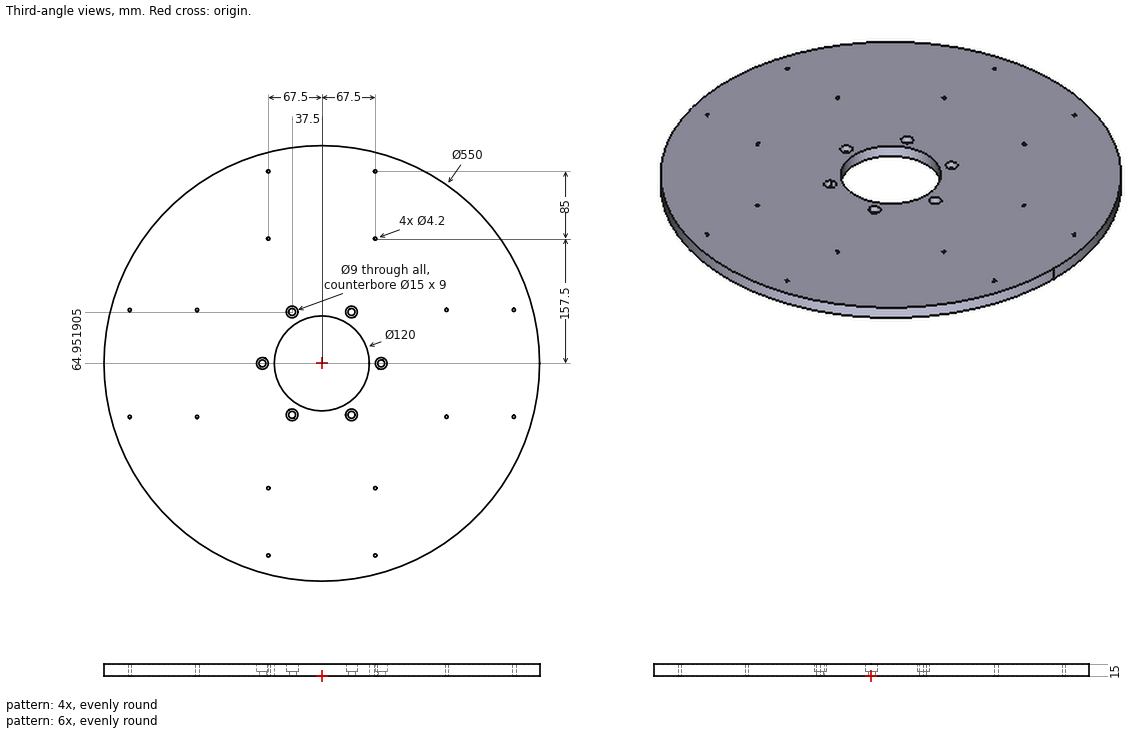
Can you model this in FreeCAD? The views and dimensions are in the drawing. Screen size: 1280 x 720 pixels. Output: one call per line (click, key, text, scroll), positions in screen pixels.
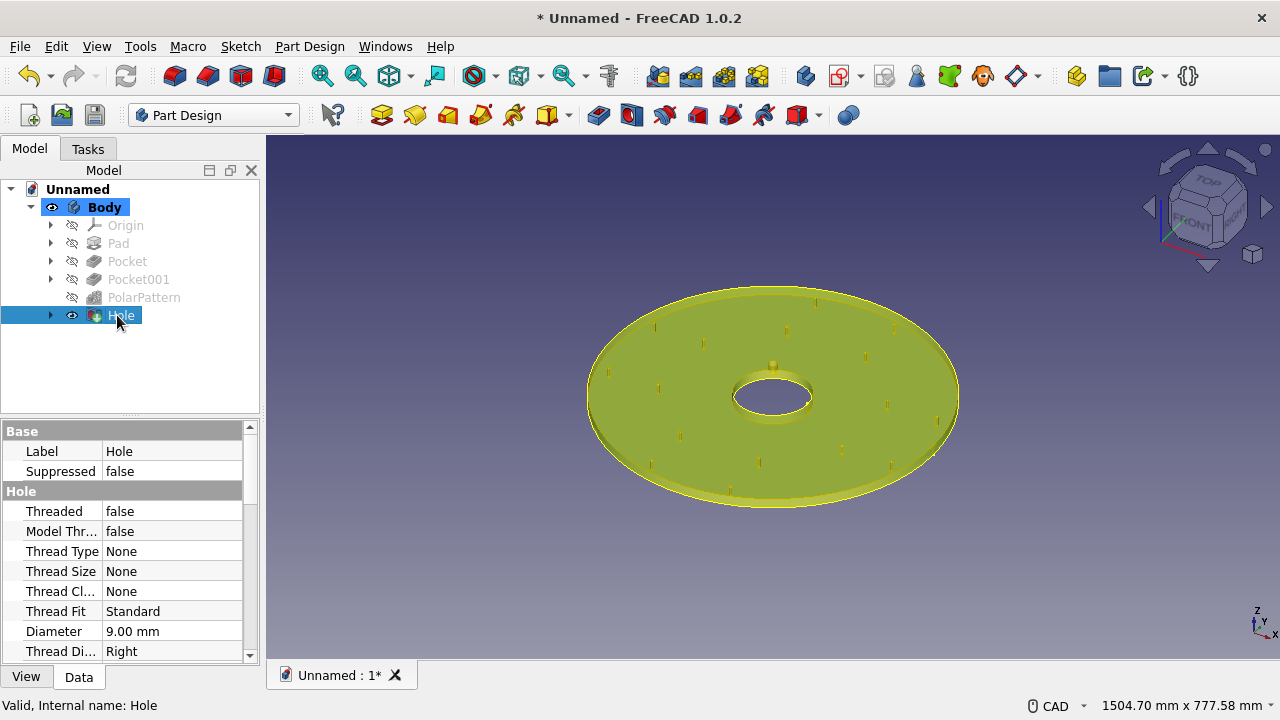
click(724, 76)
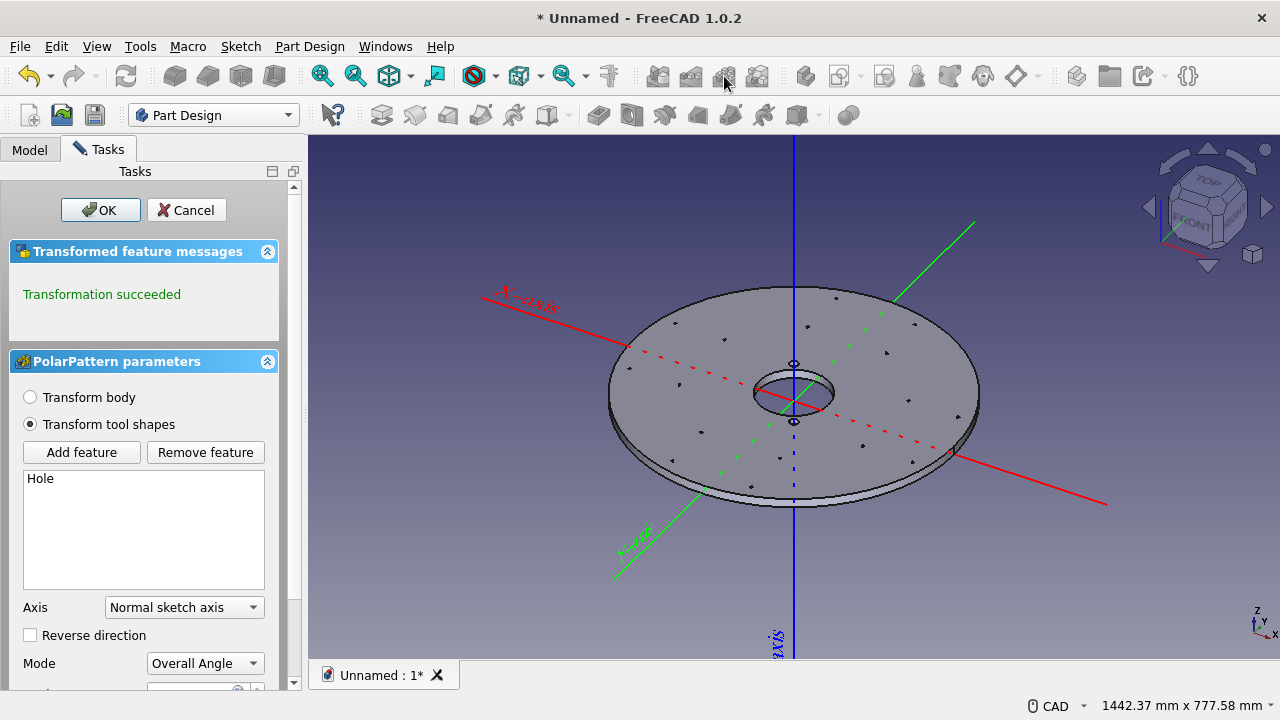
click(185, 608)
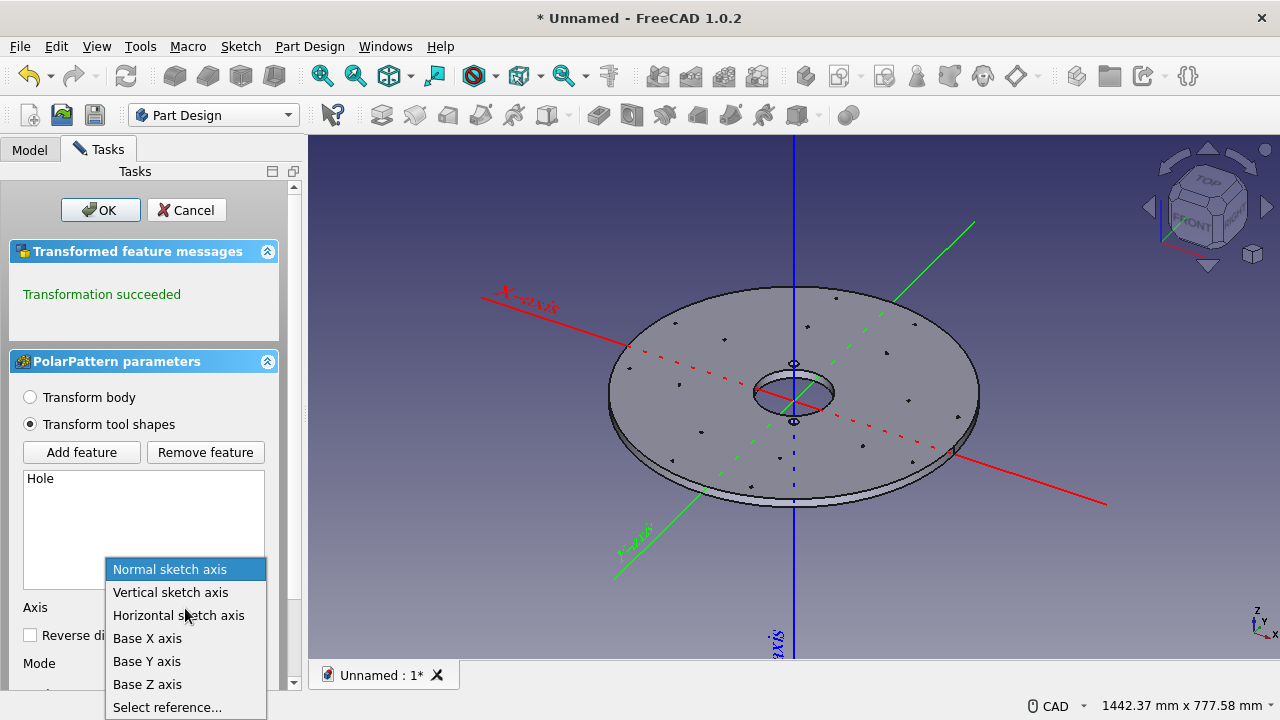
click(184, 684)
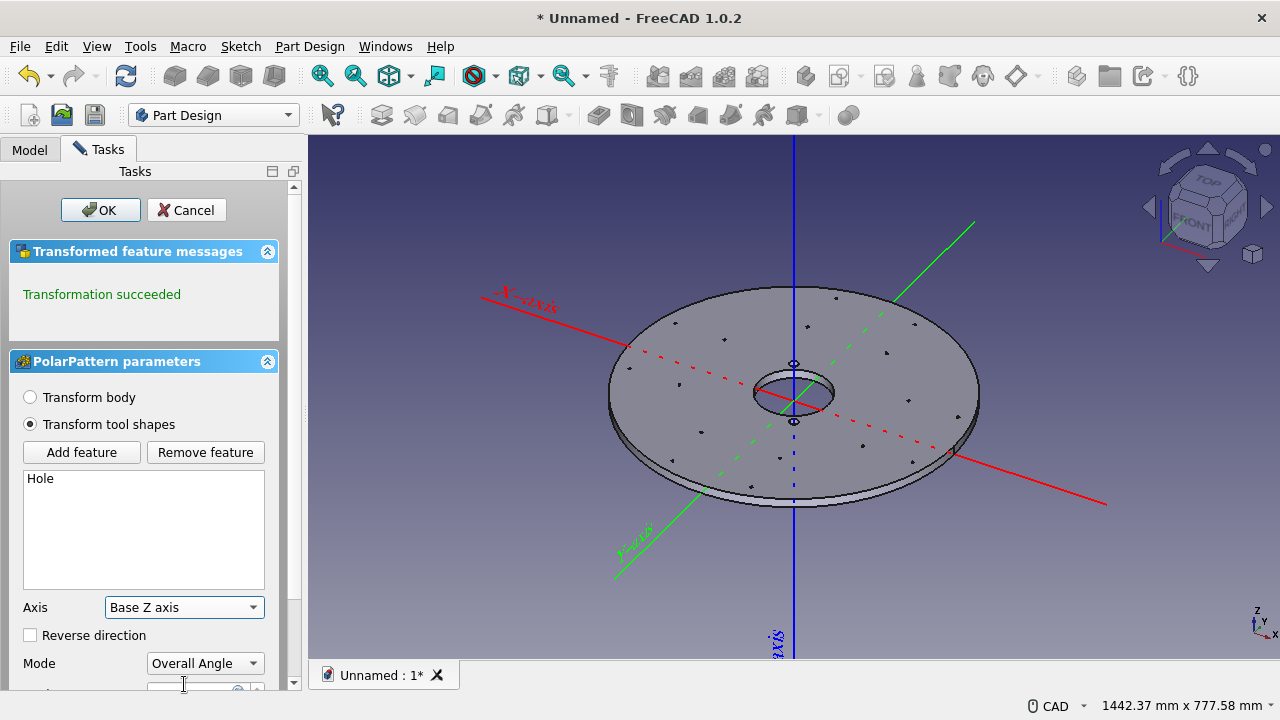
scroll(294, 436, down, 2)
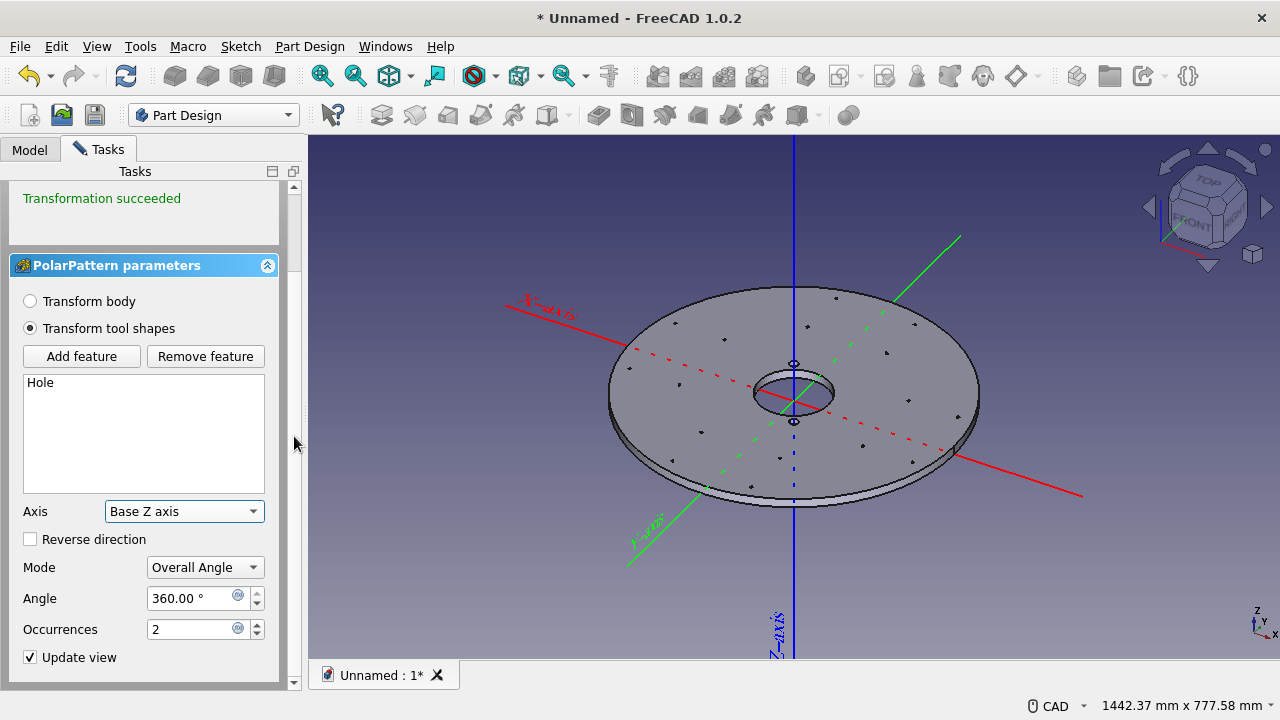
triple_click(199, 630)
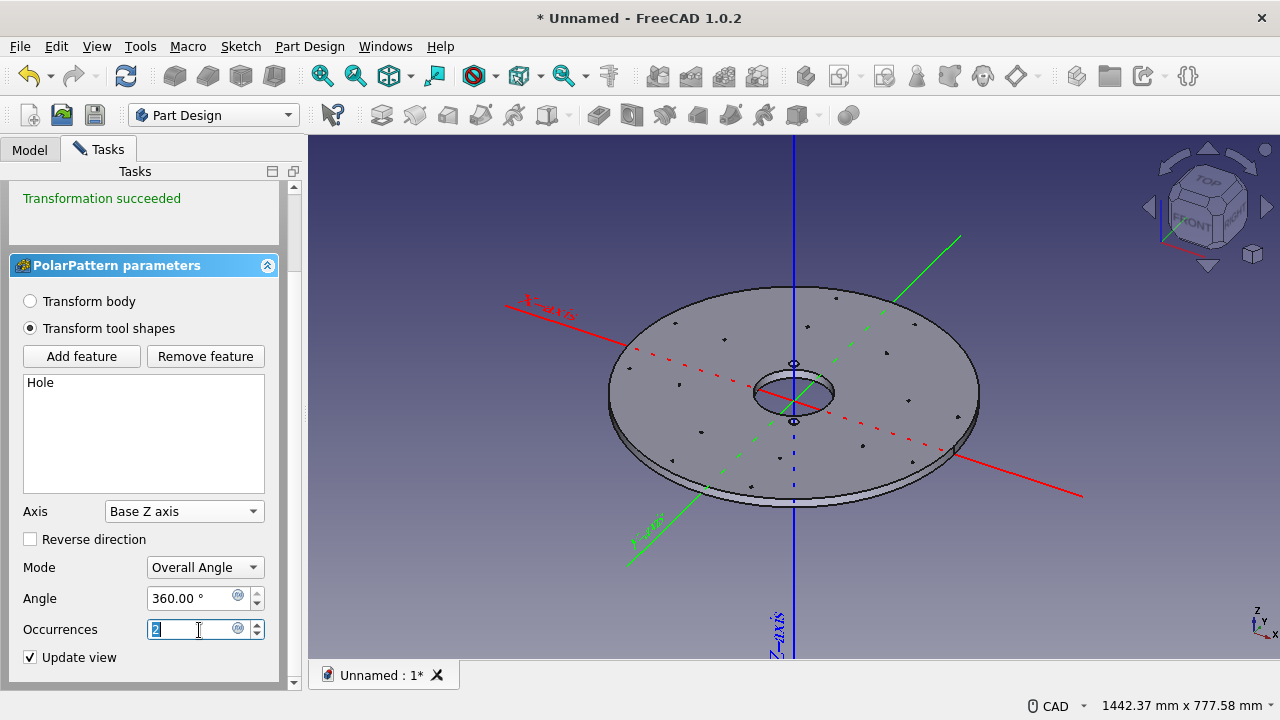
text(6)
key(Tab)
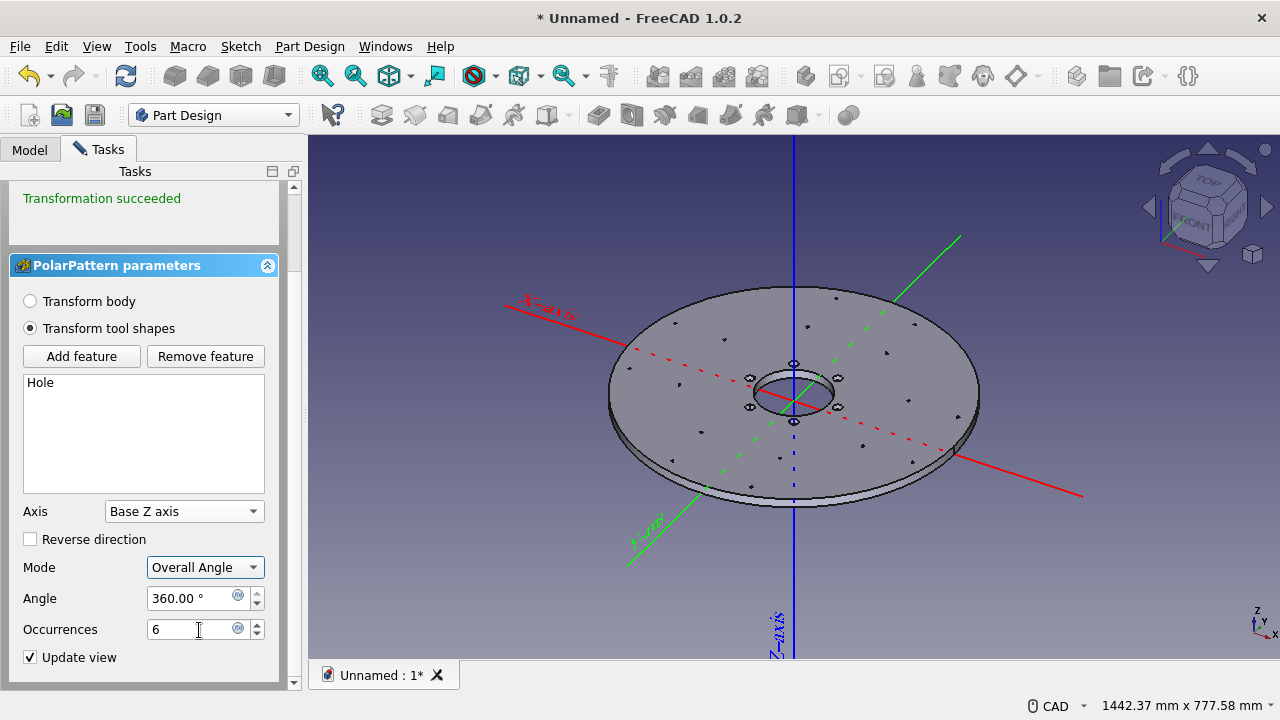
scroll(294, 436, up, 3)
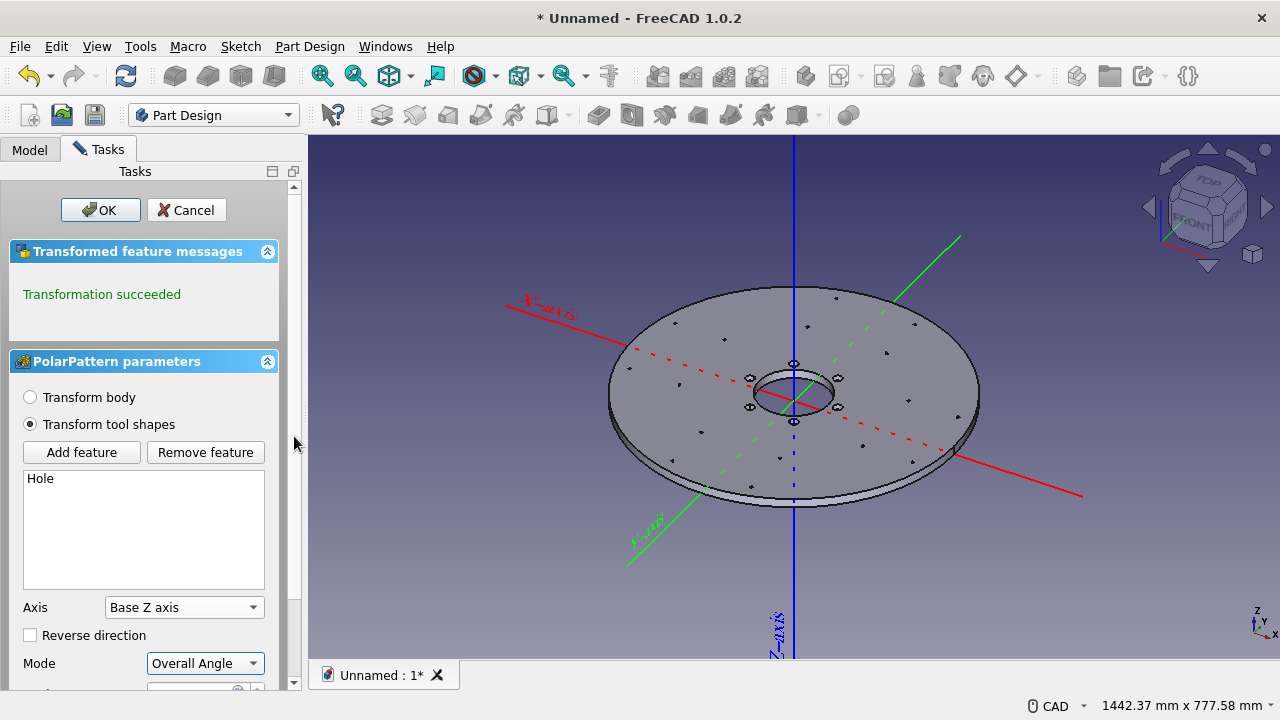
click(101, 210)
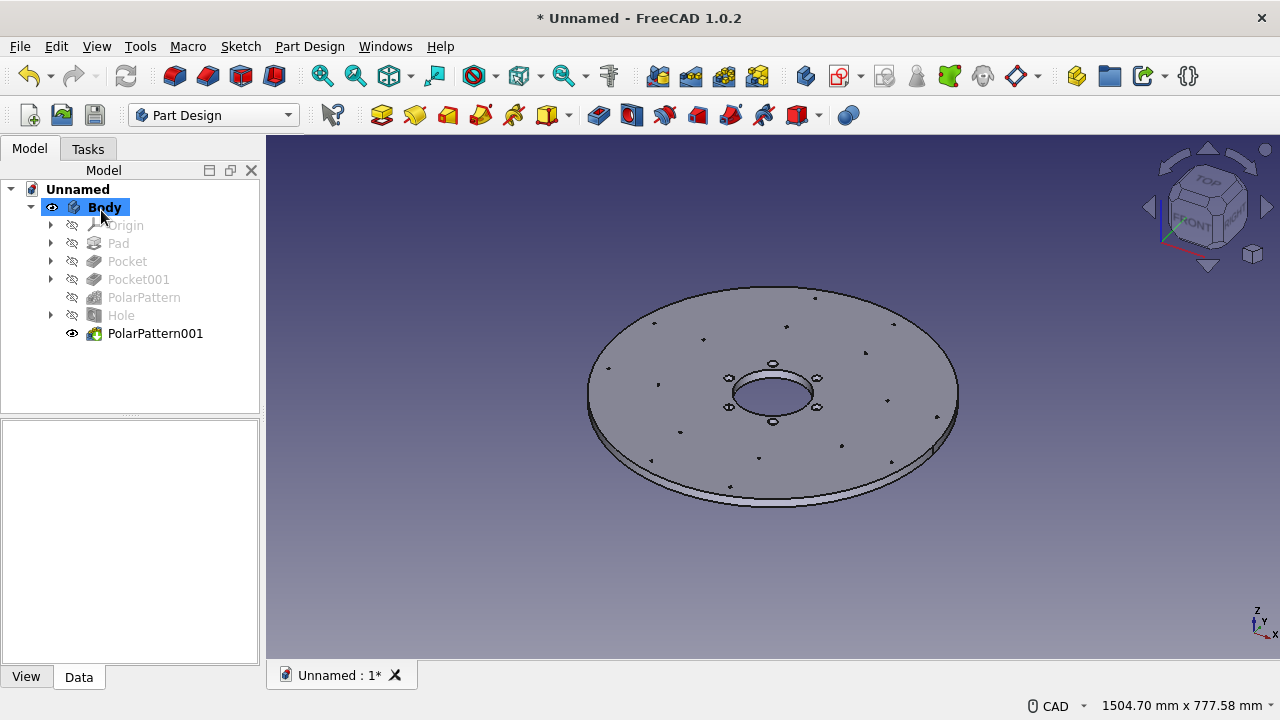
key(0)